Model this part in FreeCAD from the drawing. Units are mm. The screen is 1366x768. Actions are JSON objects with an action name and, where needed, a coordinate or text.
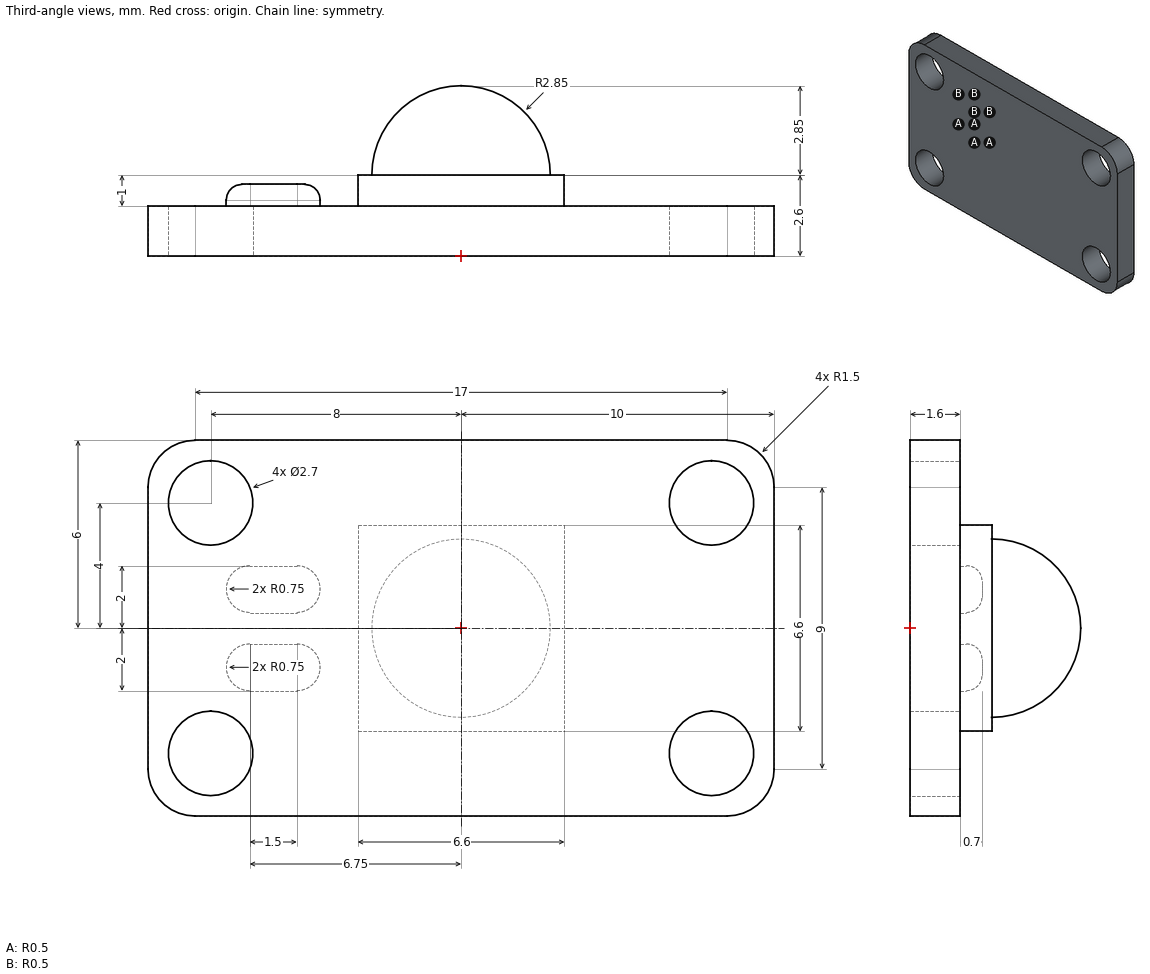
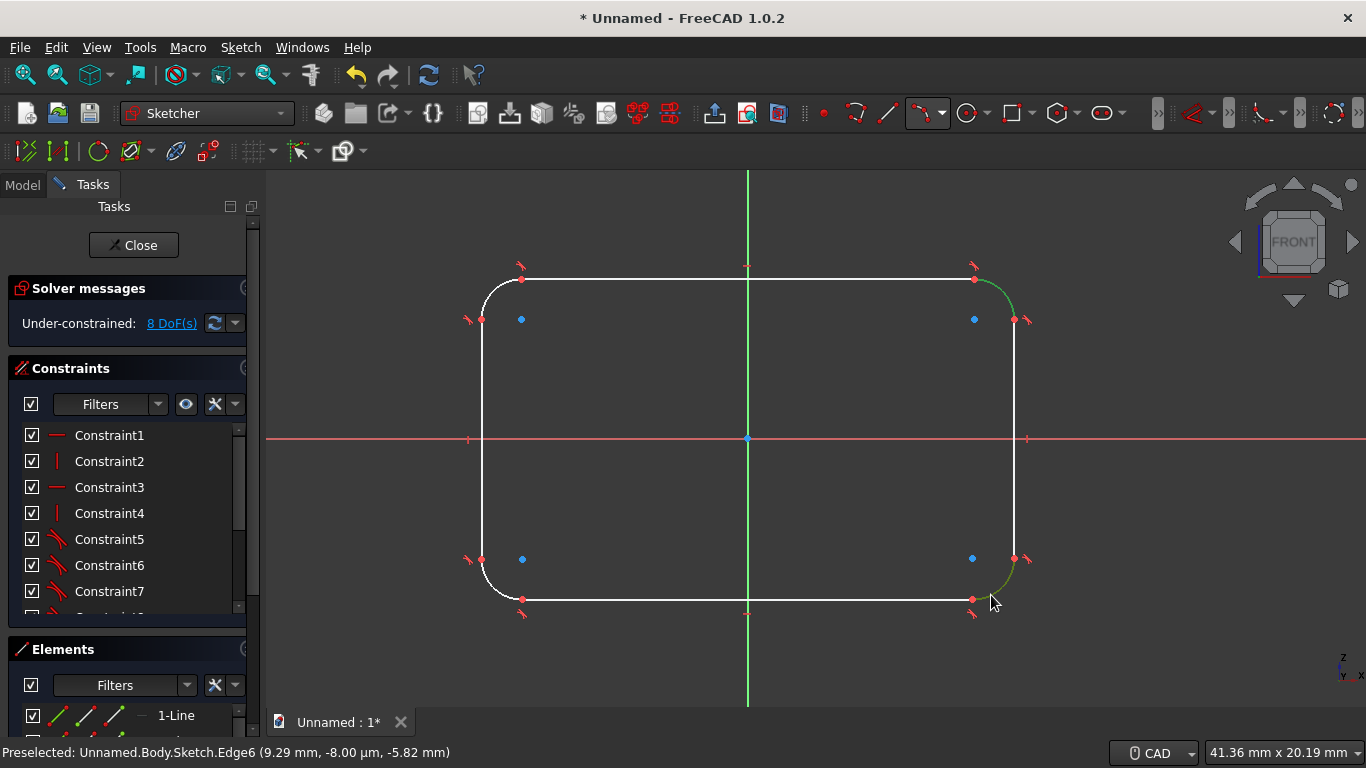
{"action": "left_click", "coordinate": [486, 578]}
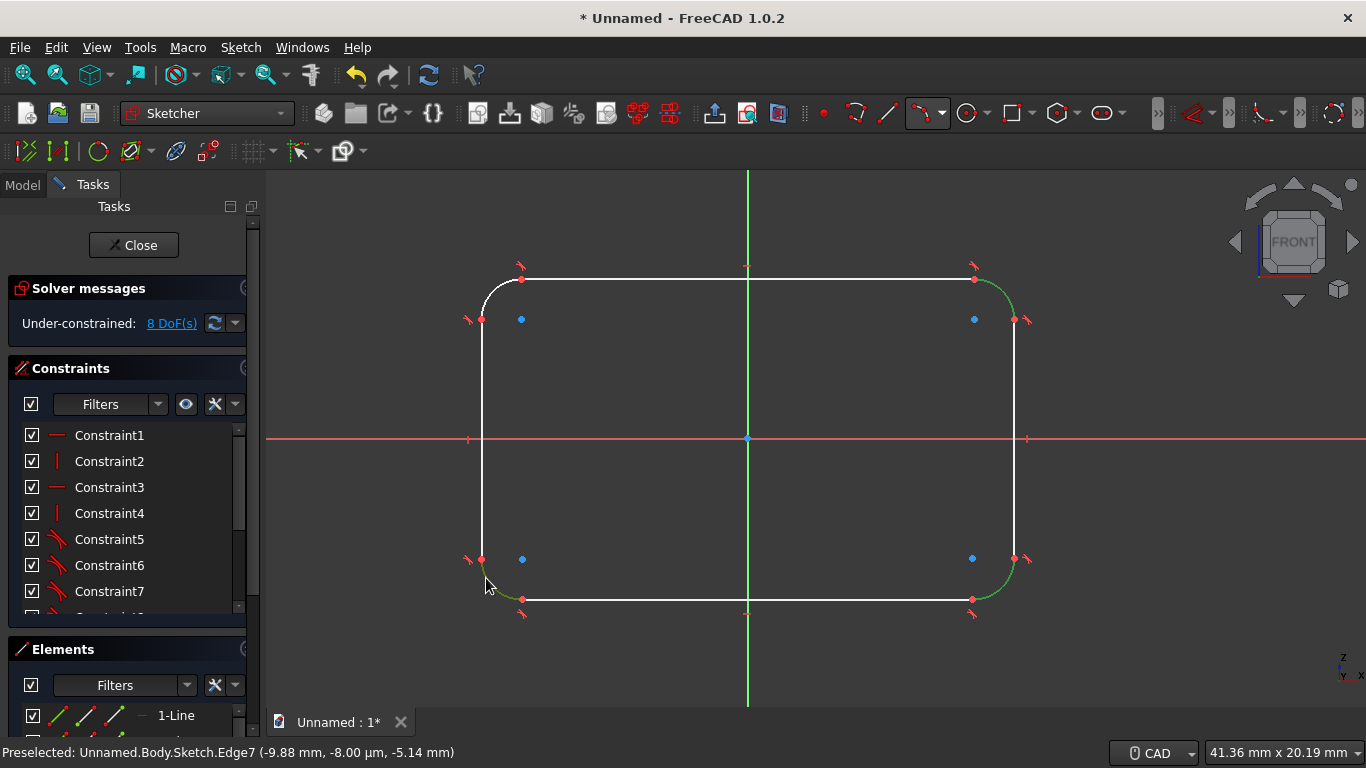
{"action": "left_click", "coordinate": [504, 284]}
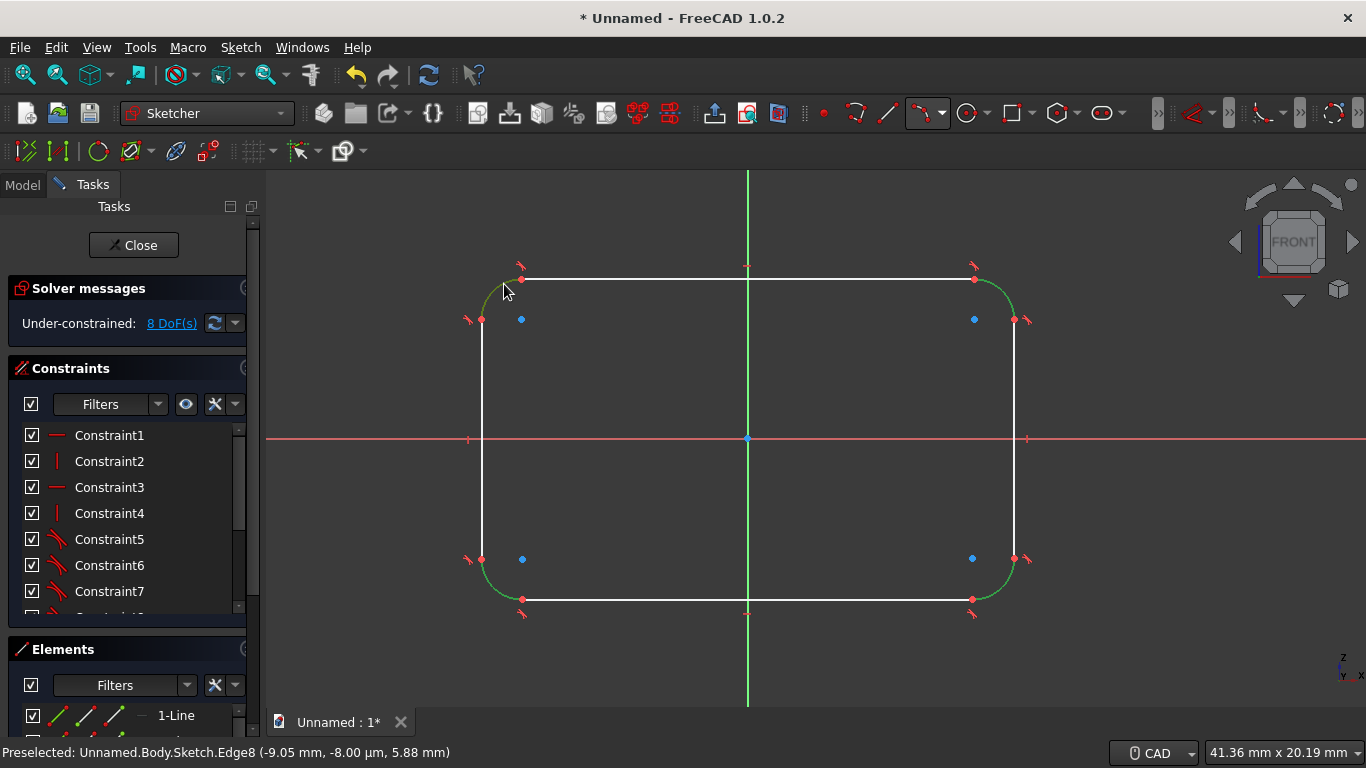
{"action": "key", "text": "e"}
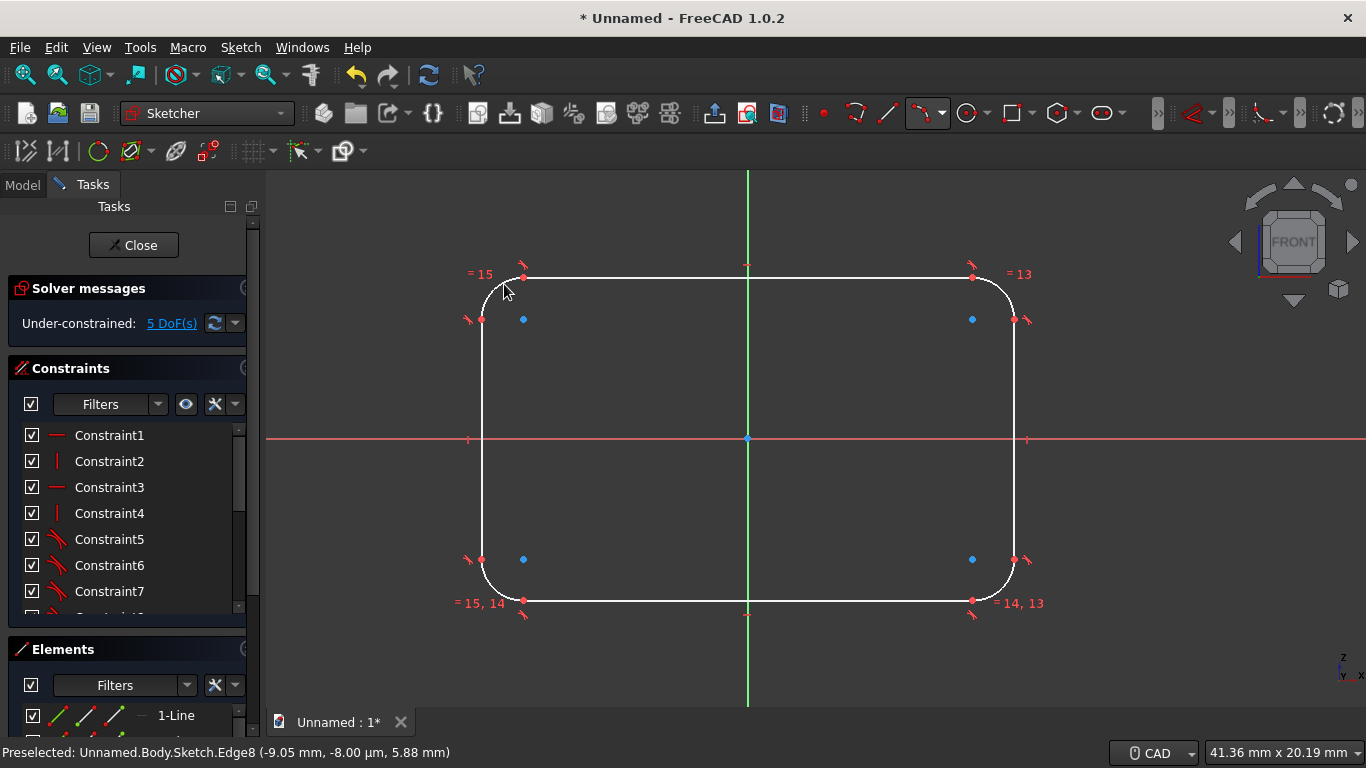
{"action": "left_click", "coordinate": [1192, 114]}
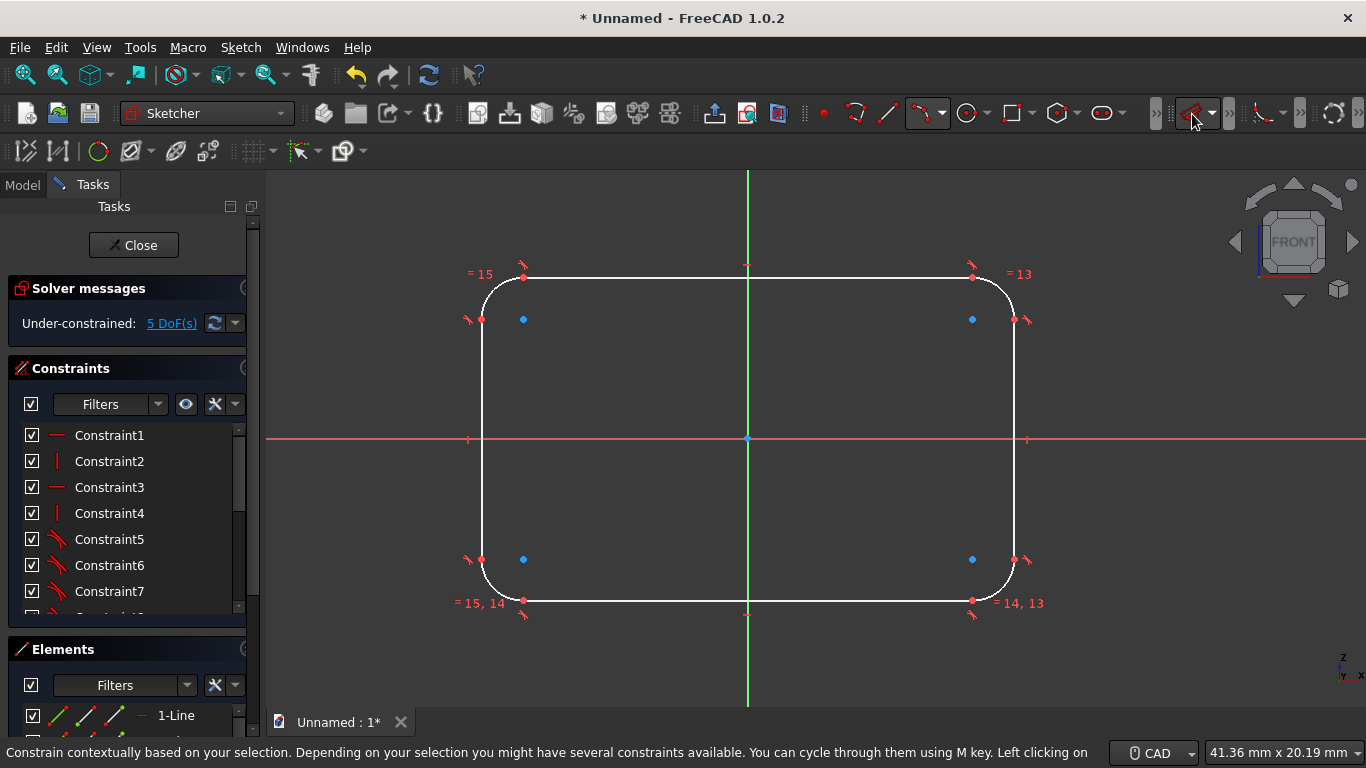
{"action": "left_click", "coordinate": [1010, 301]}
{"action": "left_click", "coordinate": [1039, 287]}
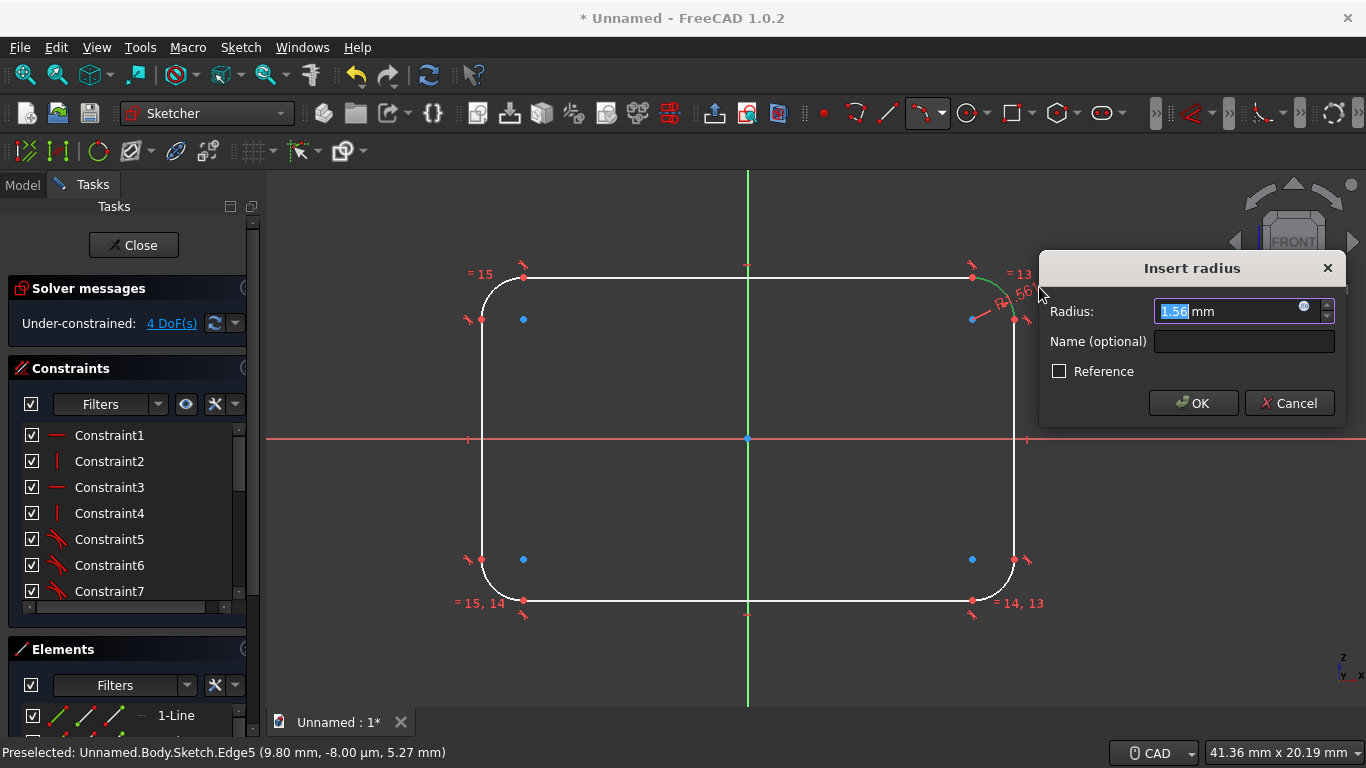
{"action": "type", "text": "1.5"}
{"action": "key", "text": "Return"}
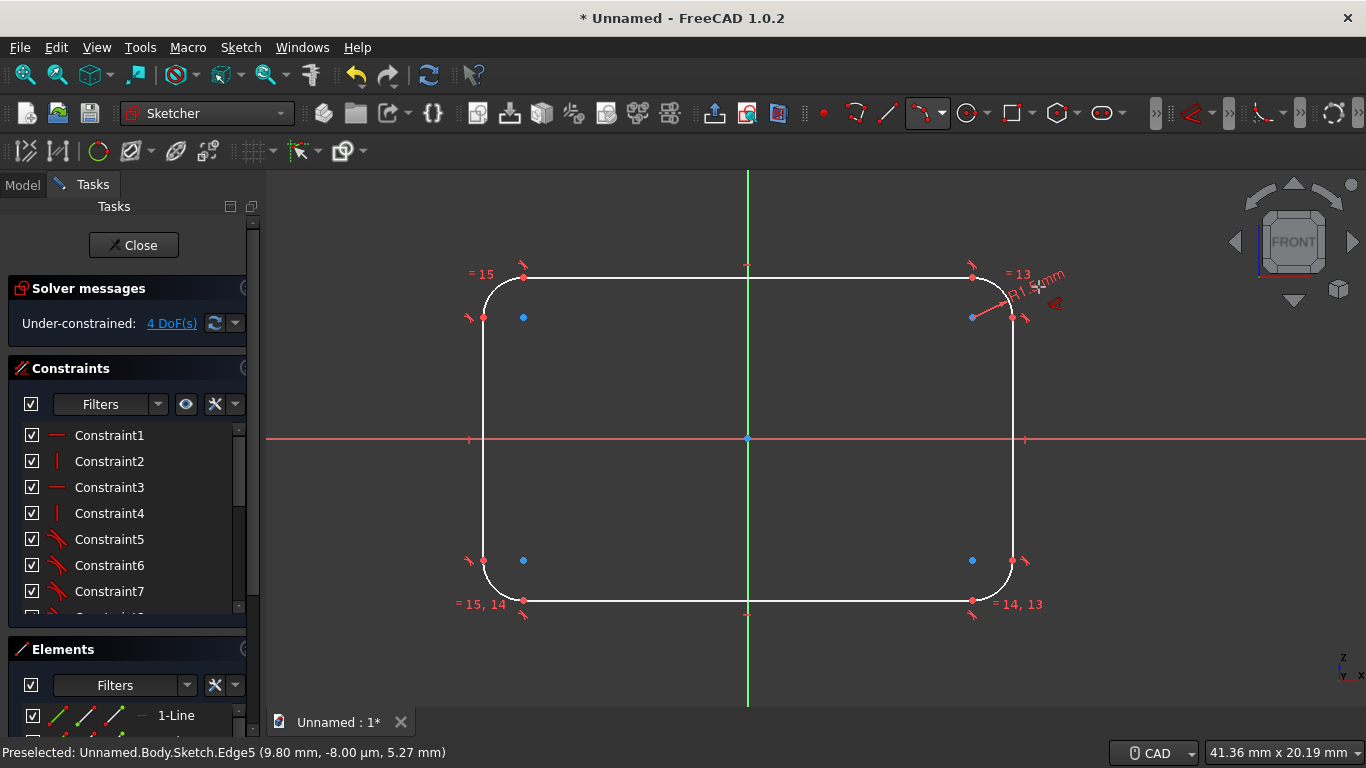
{"action": "left_click", "coordinate": [1013, 391]}
{"action": "left_click", "coordinate": [1047, 383]}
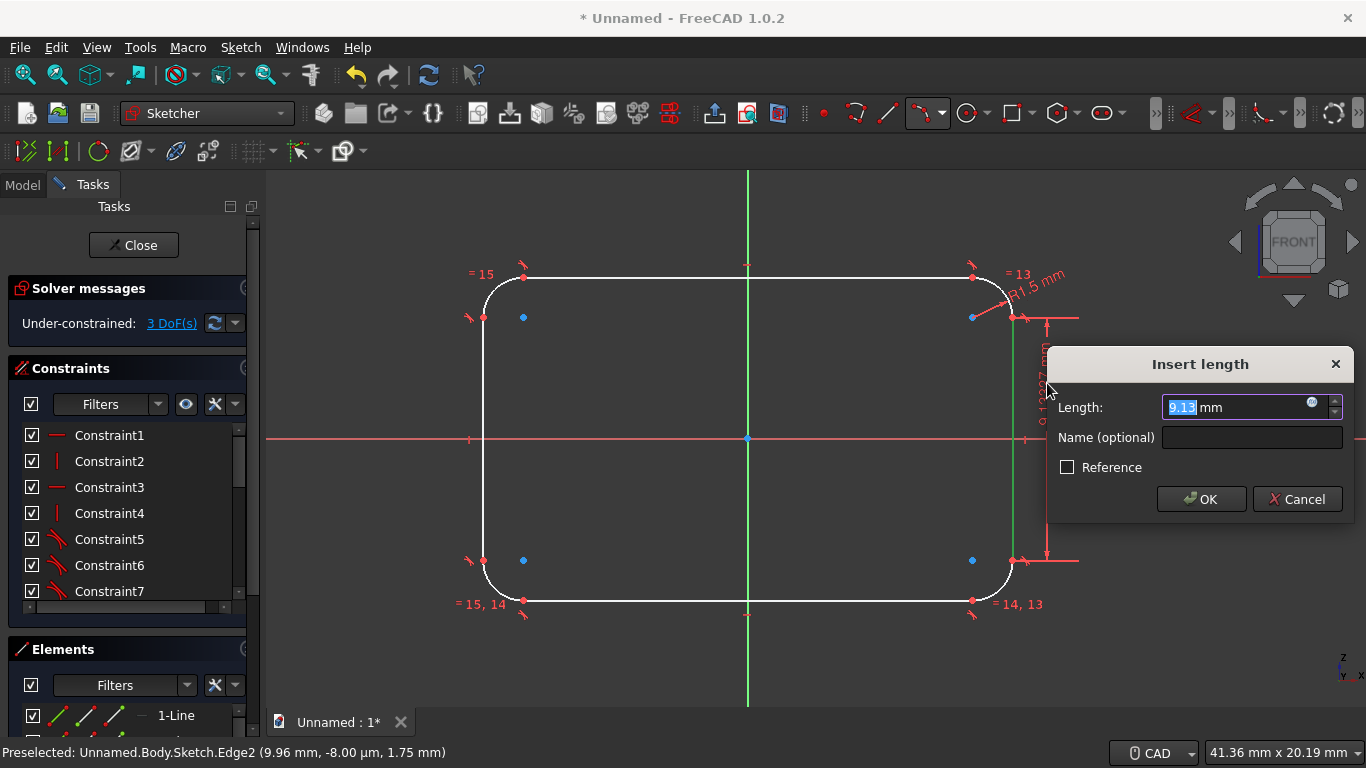
{"action": "type", "text": "9"}
{"action": "key", "text": "Return"}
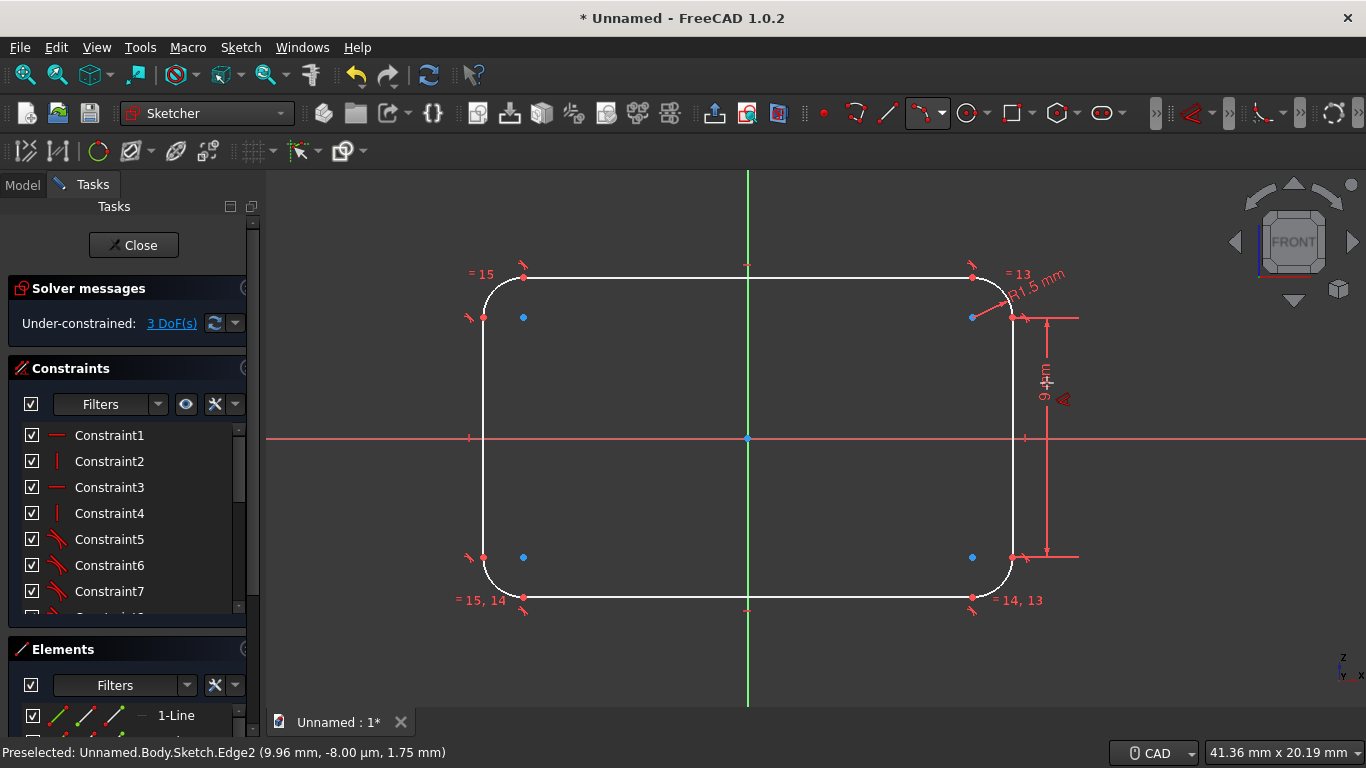
{"action": "left_click", "coordinate": [658, 278]}
{"action": "left_click", "coordinate": [645, 244]}